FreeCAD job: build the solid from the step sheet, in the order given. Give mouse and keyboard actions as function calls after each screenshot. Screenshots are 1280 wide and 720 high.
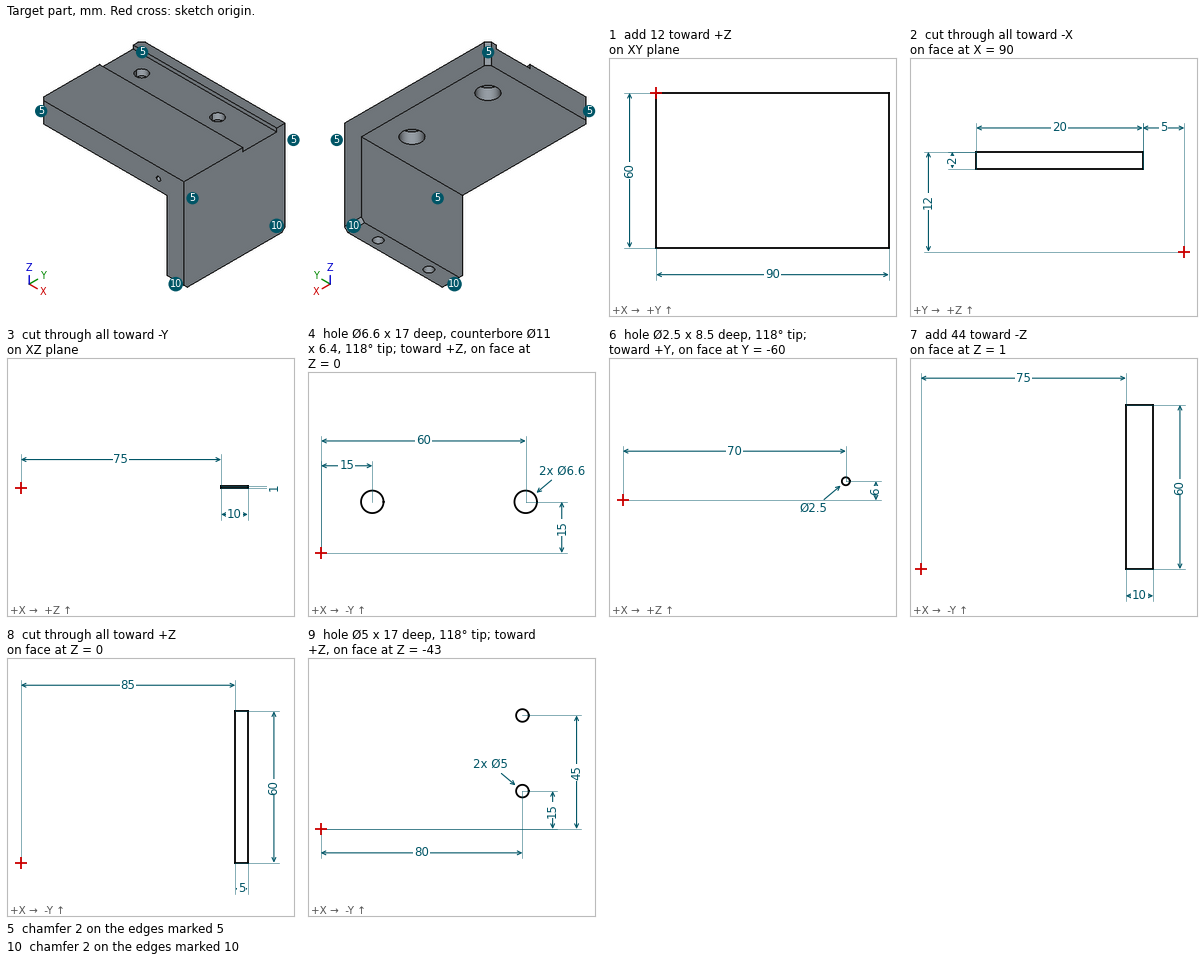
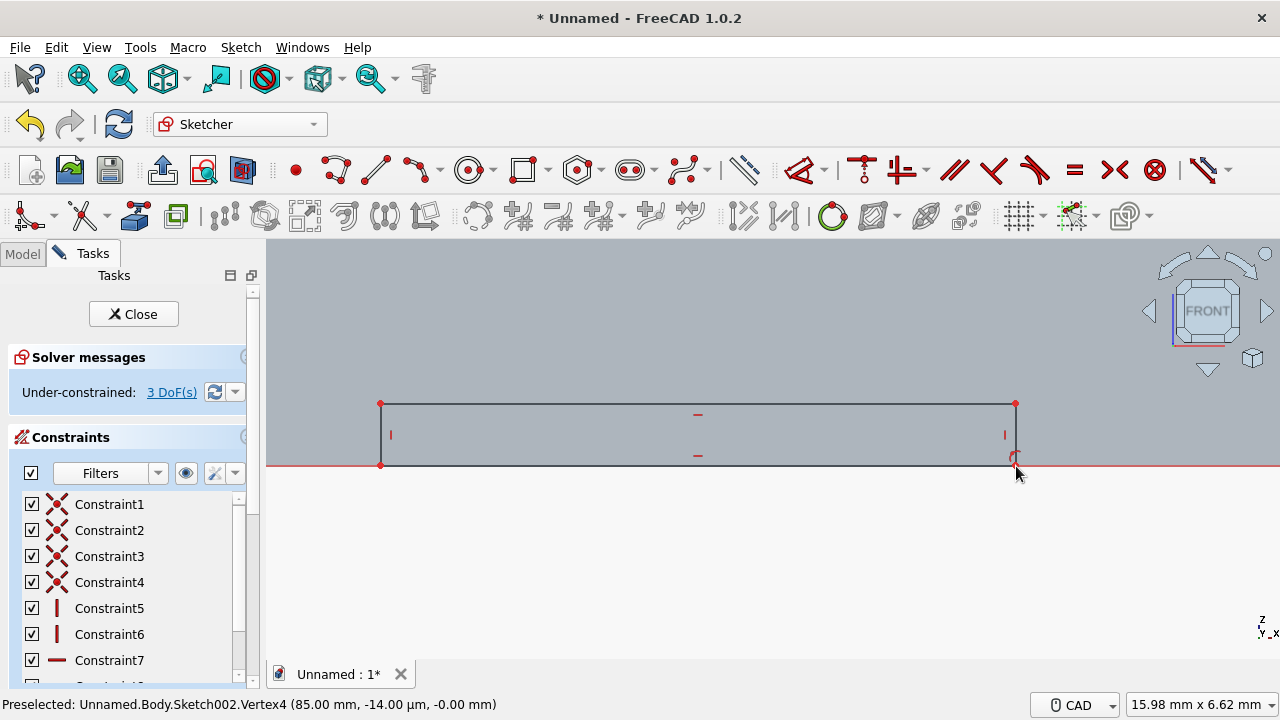
key(d)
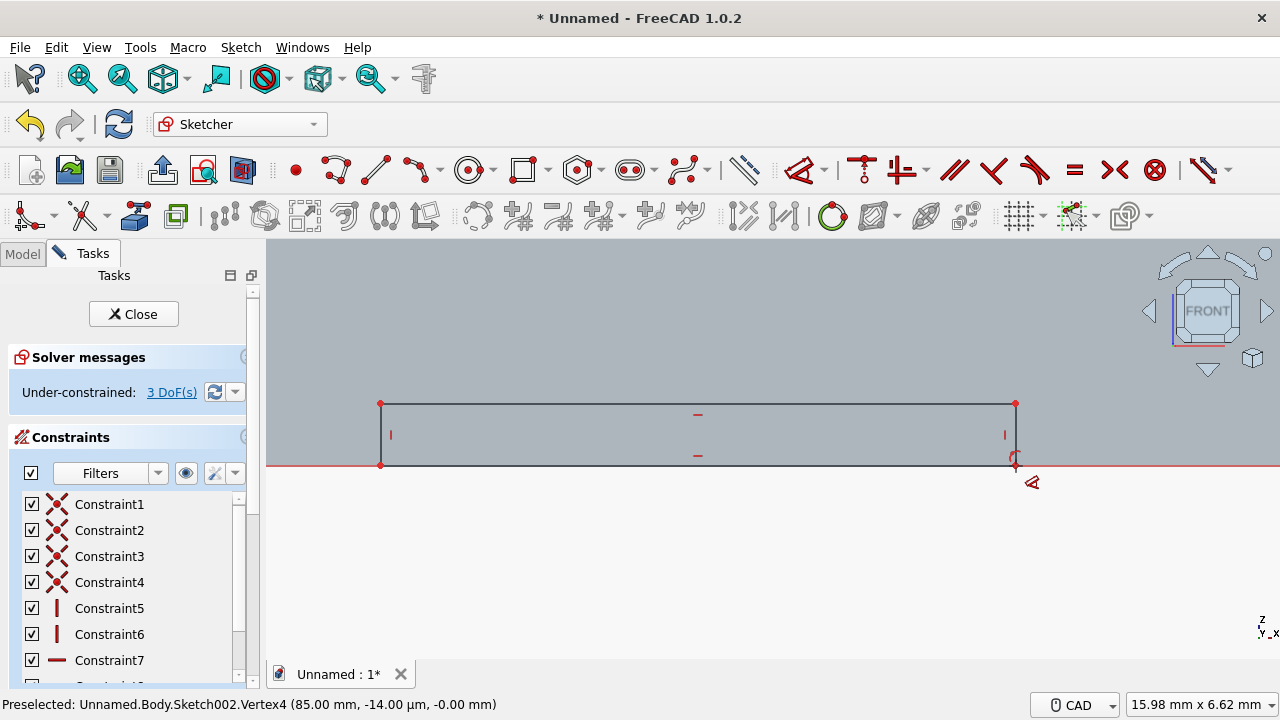
click(381, 423)
click(347, 435)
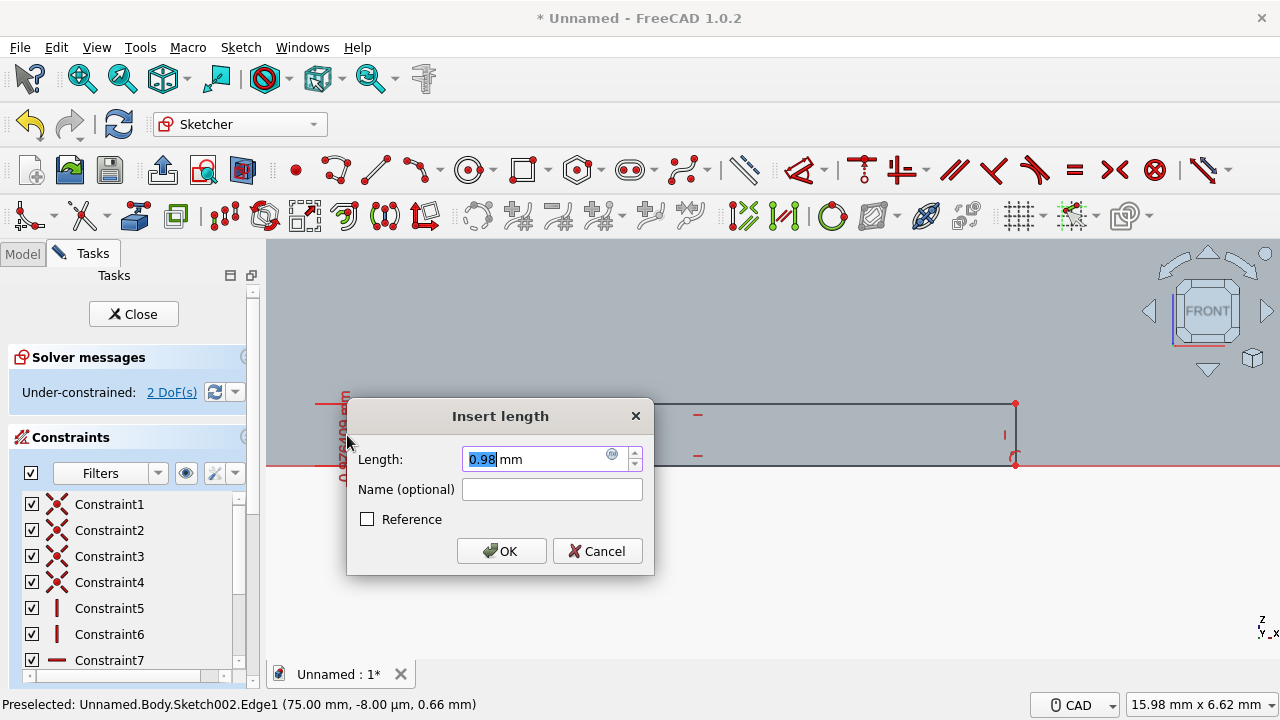
text(1)
key(Return)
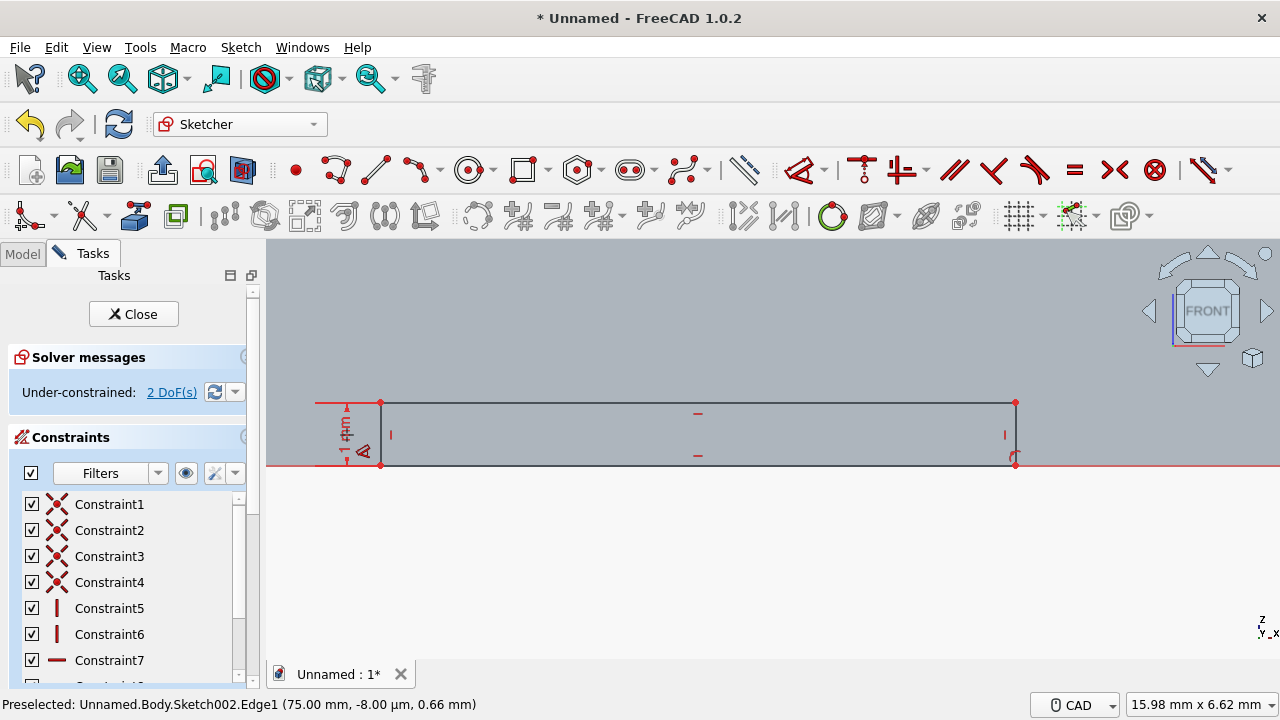
click(571, 466)
click(698, 500)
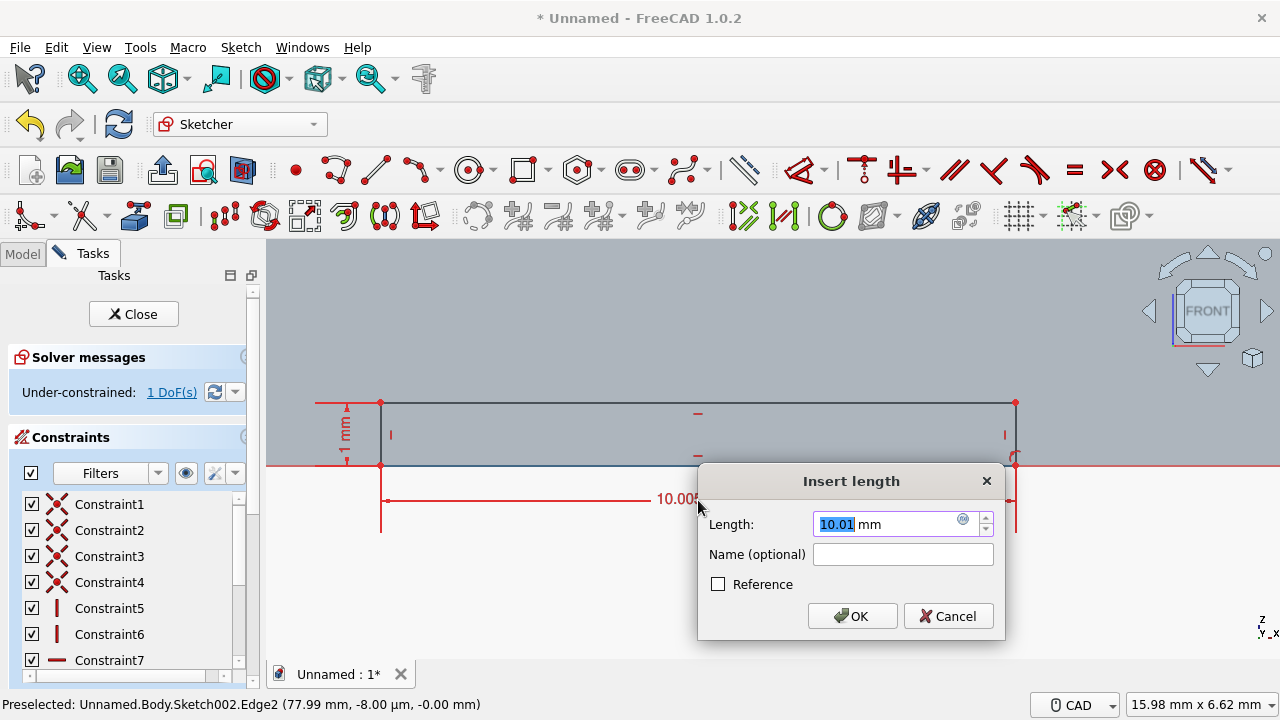
text(10)
key(Return)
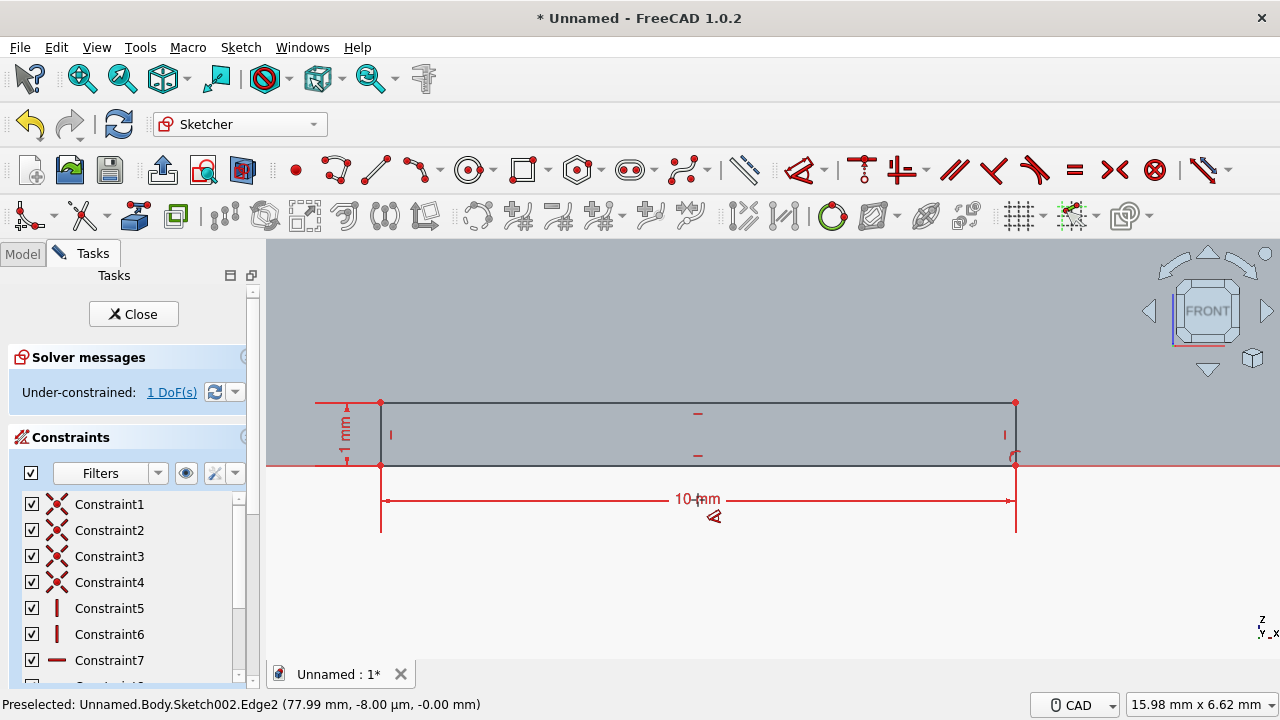
click(381, 403)
click(337, 500)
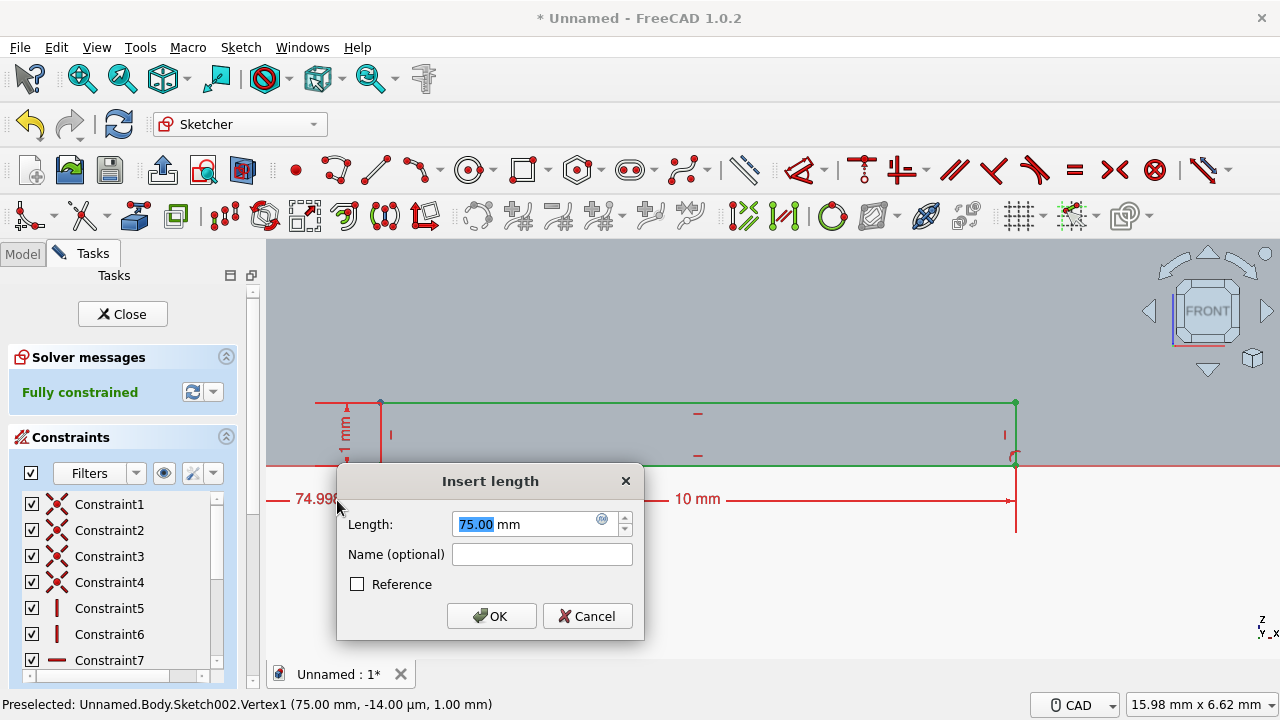
text(75)
key(Return)
key(Escape)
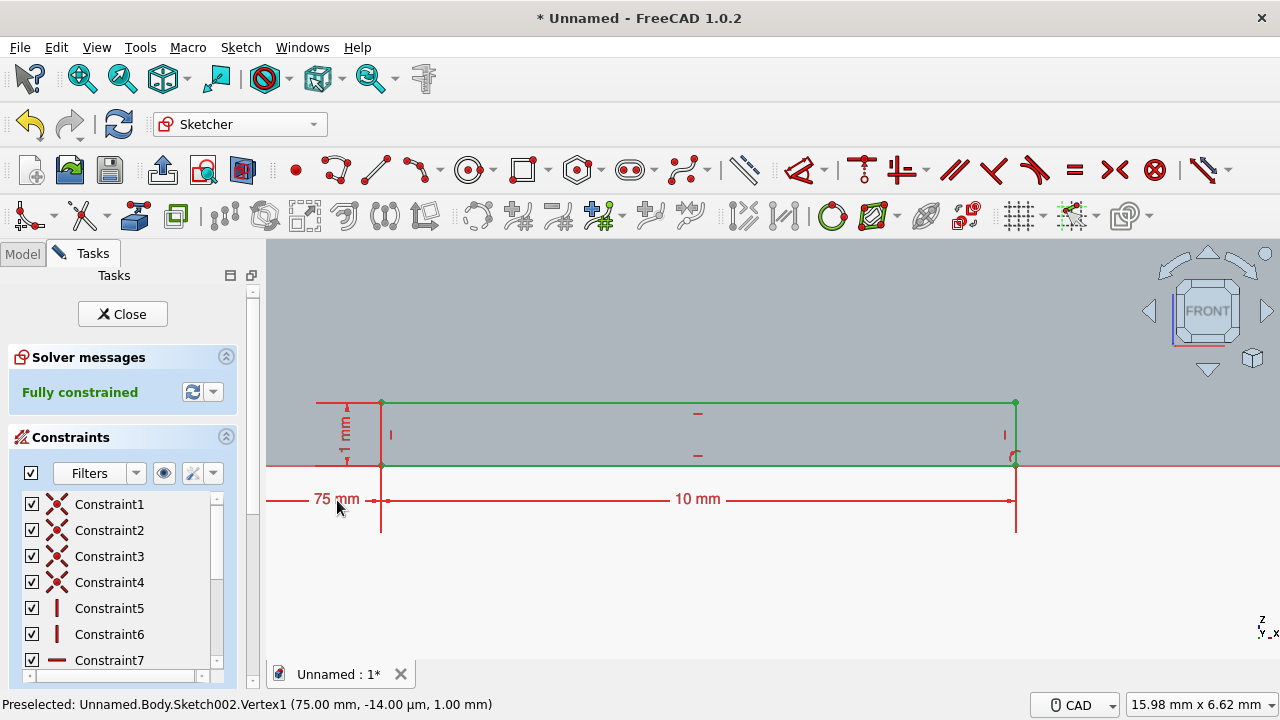
click(123, 314)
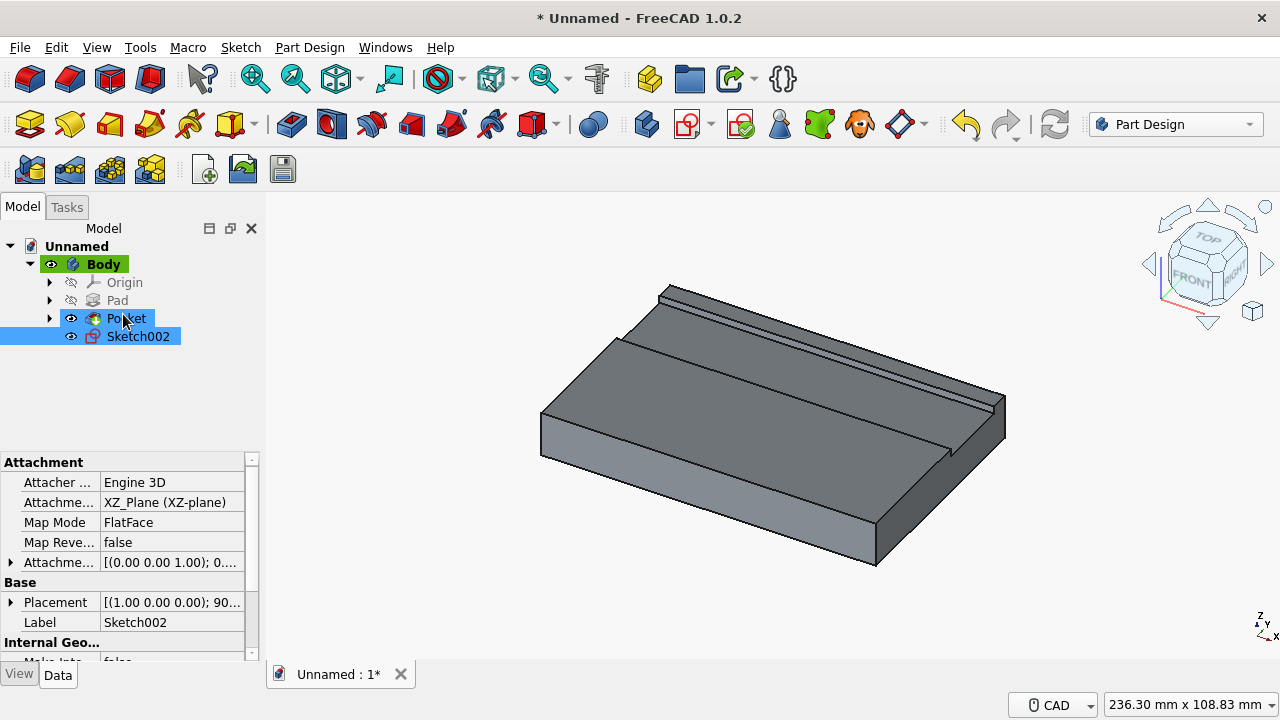
click(292, 124)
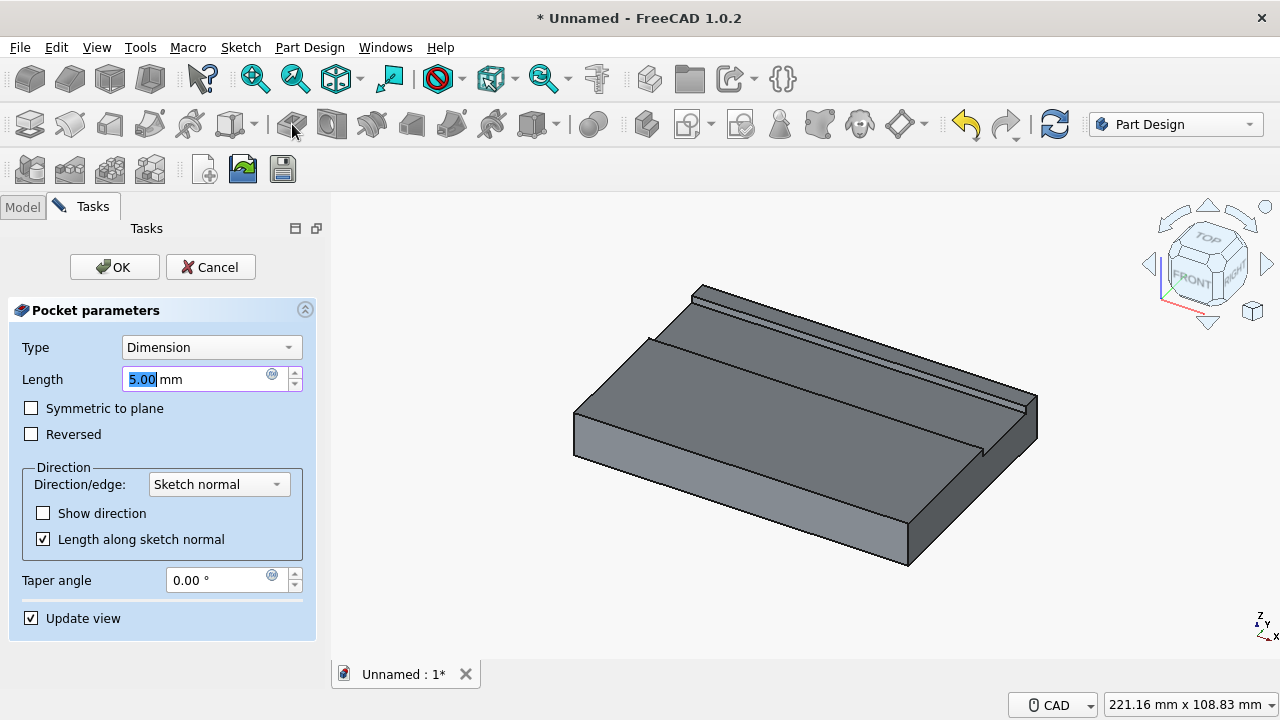
click(212, 348)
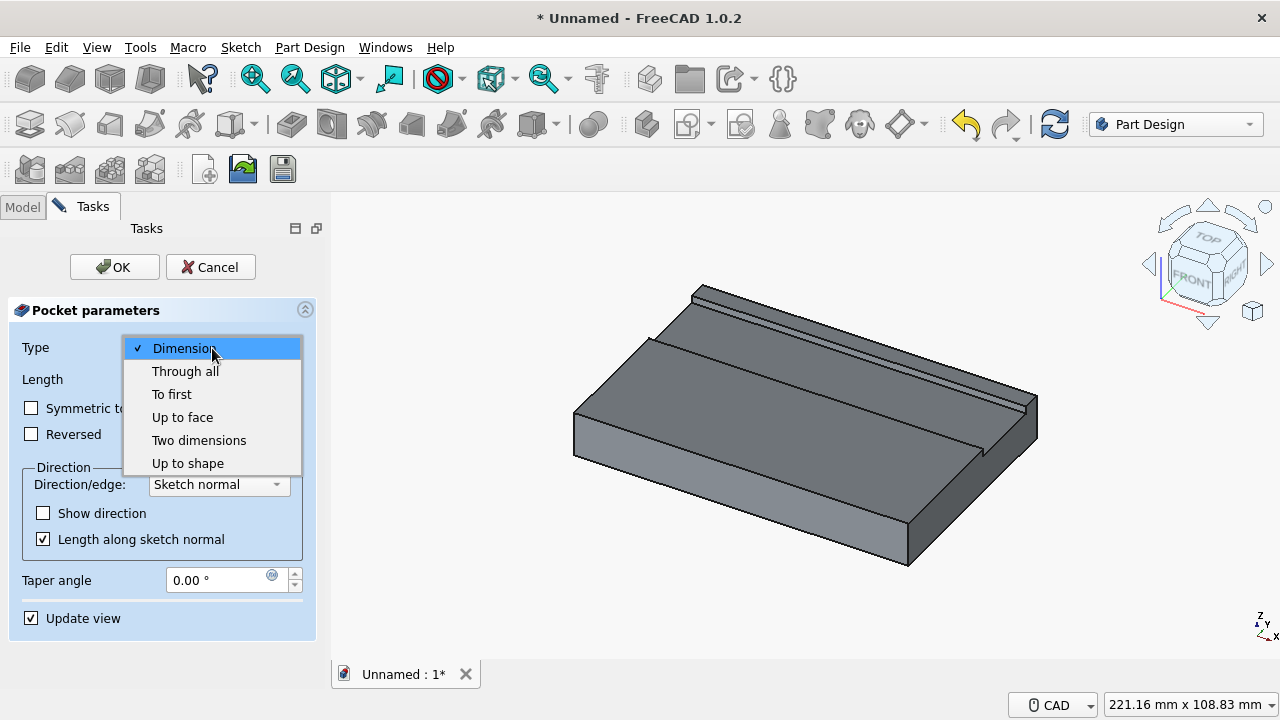
click(212, 372)